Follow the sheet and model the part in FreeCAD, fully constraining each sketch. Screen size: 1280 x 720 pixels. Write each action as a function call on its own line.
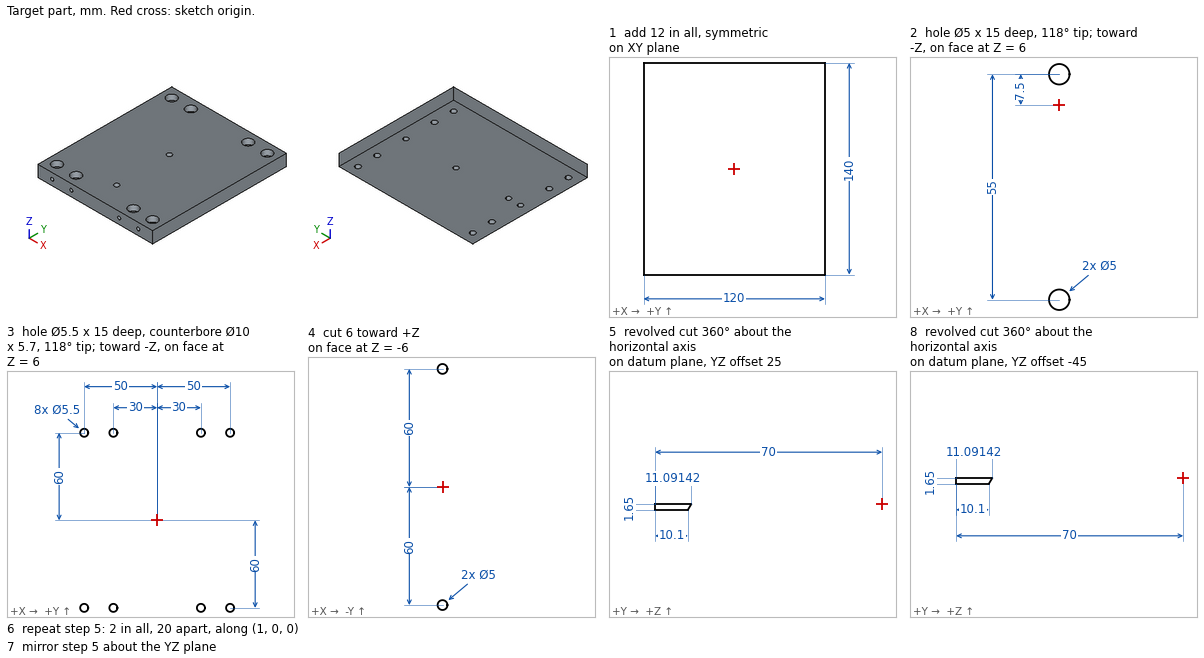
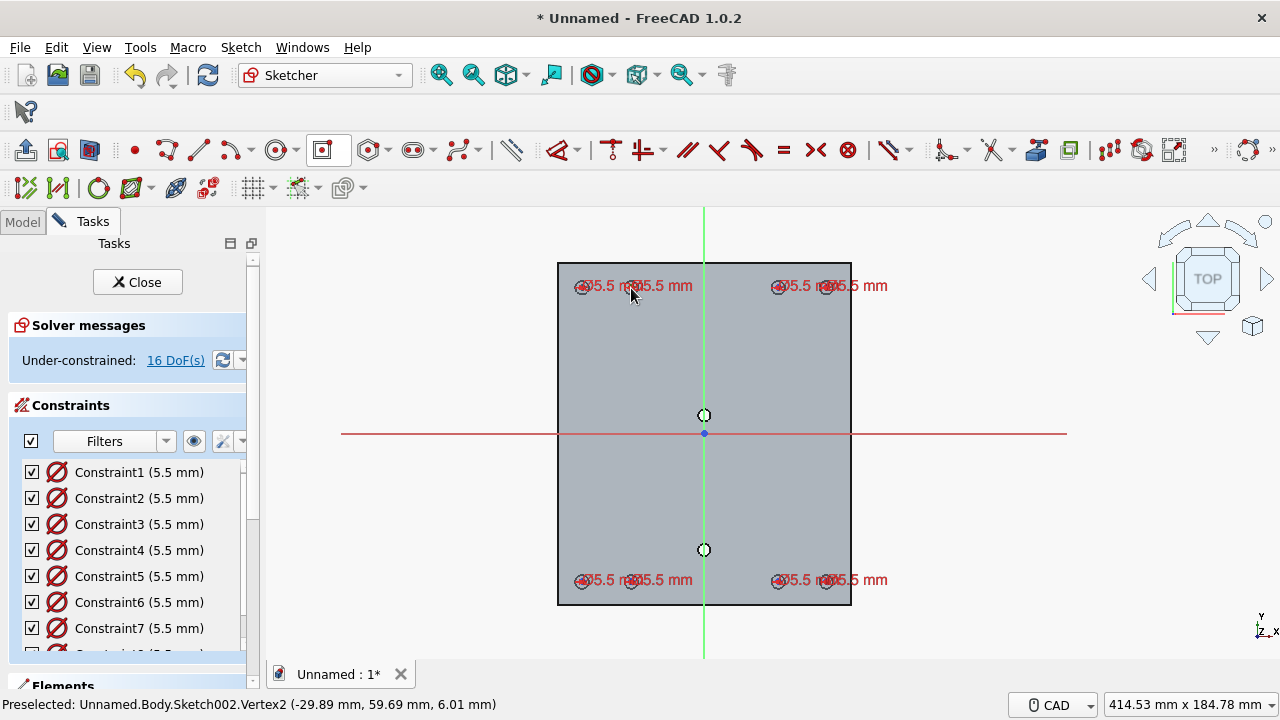
key(h)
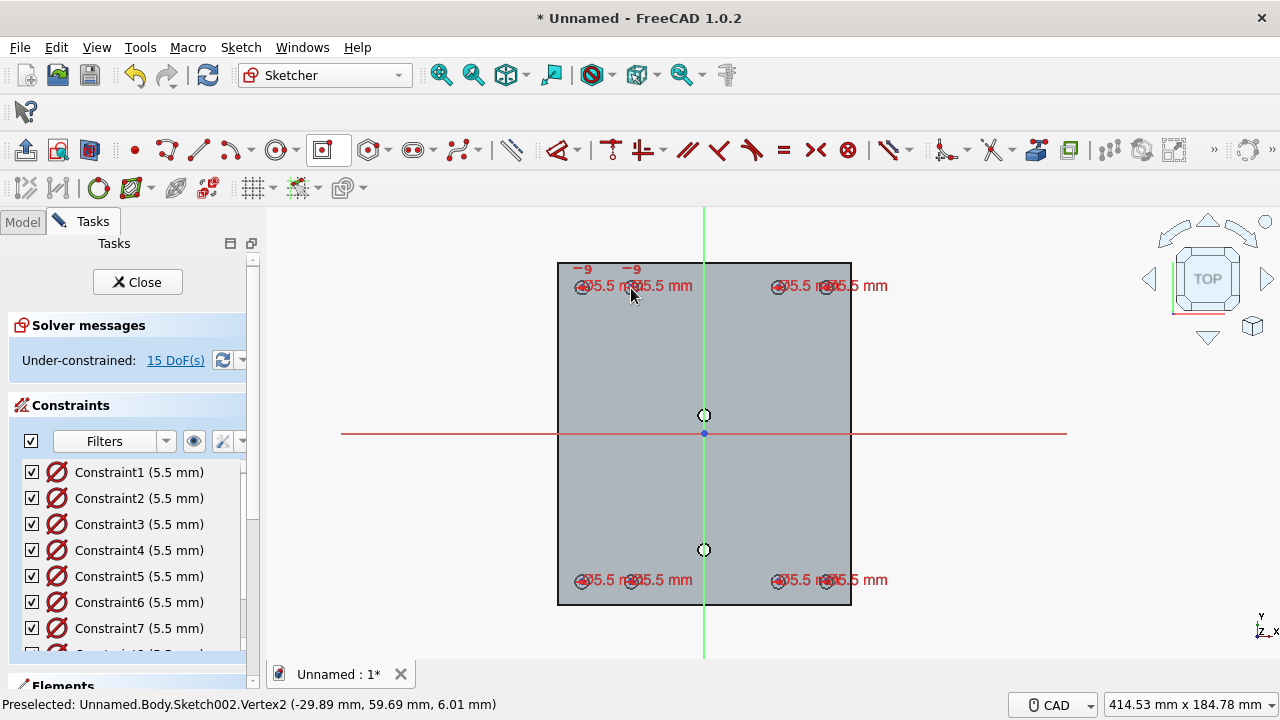
click(631, 288)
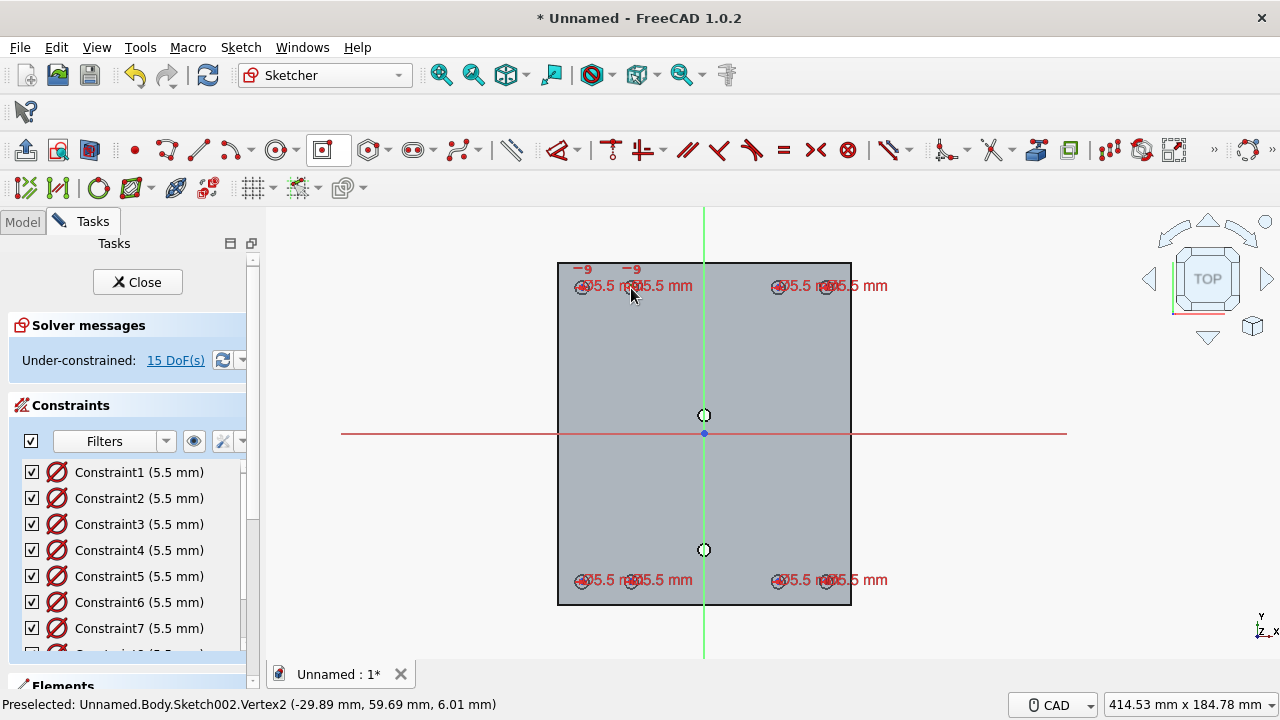
click(778, 288)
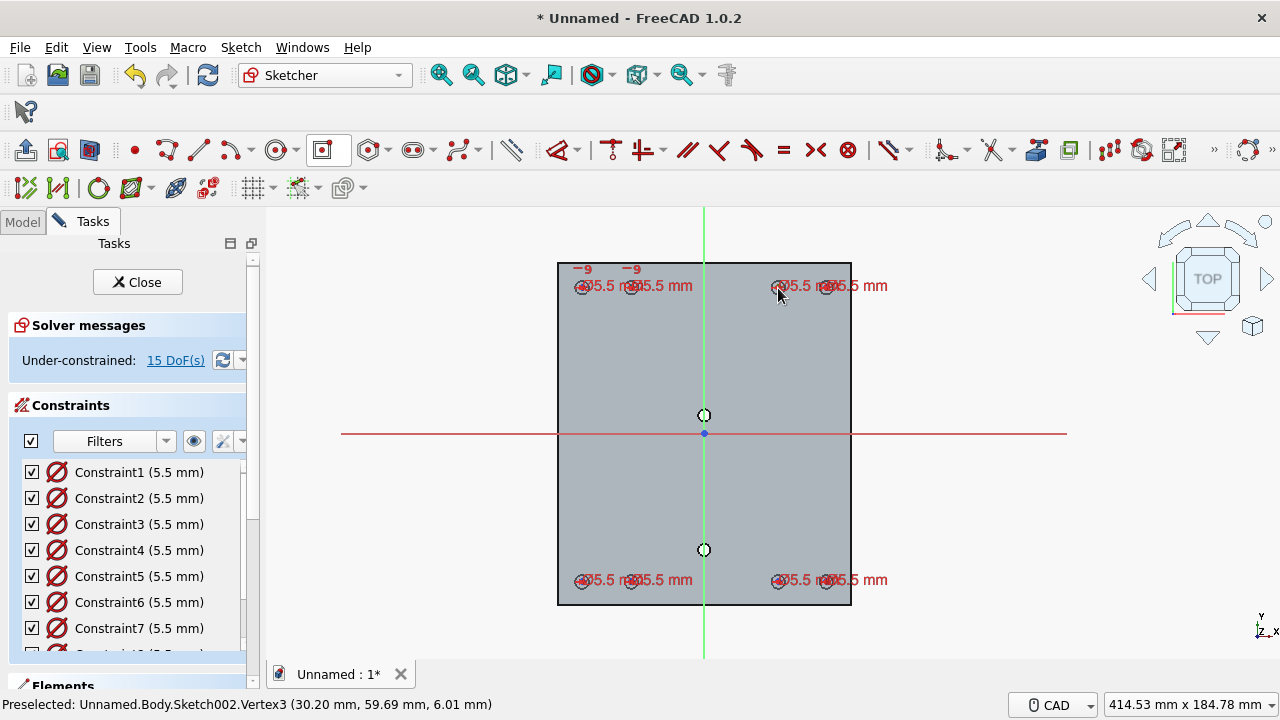
key(h)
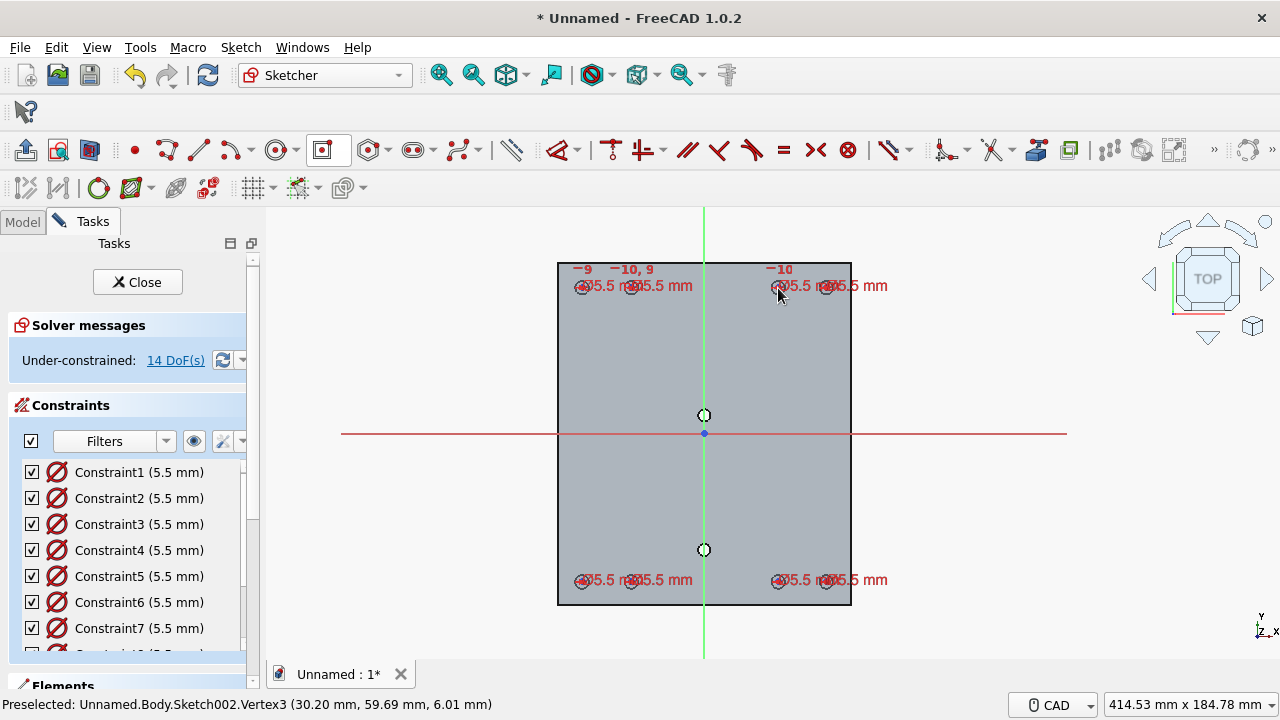
click(778, 288)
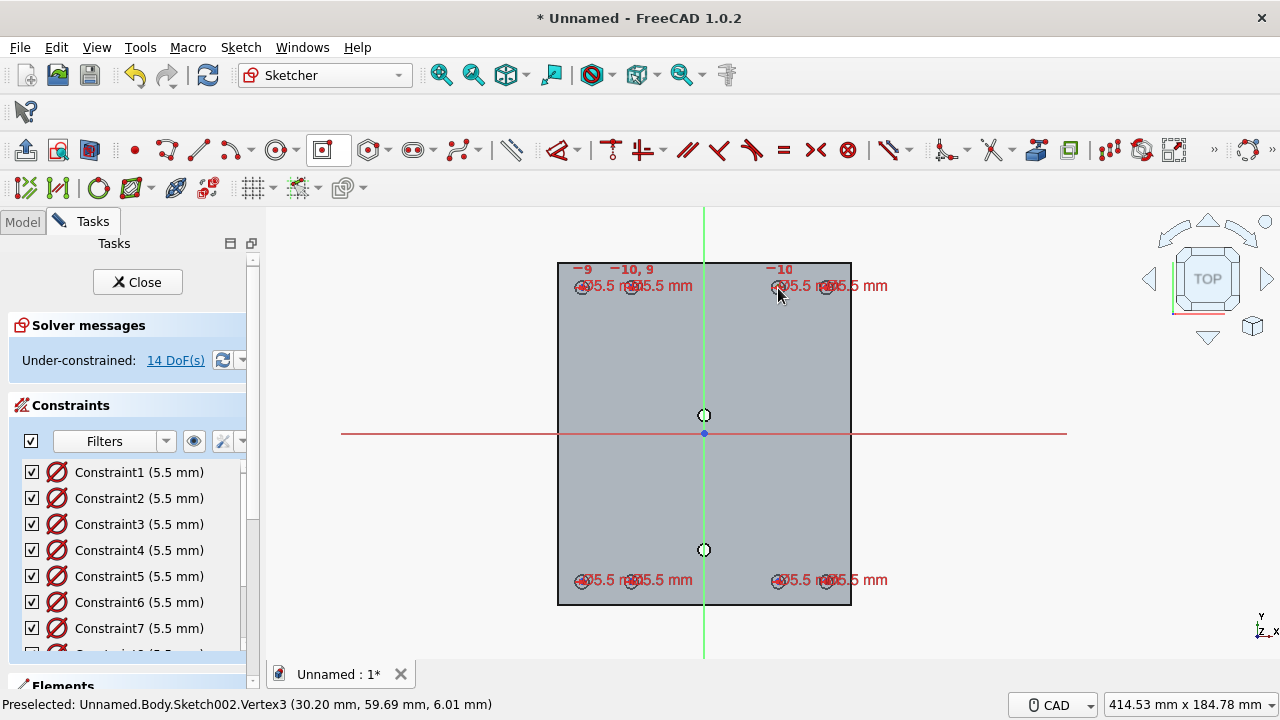
click(826, 288)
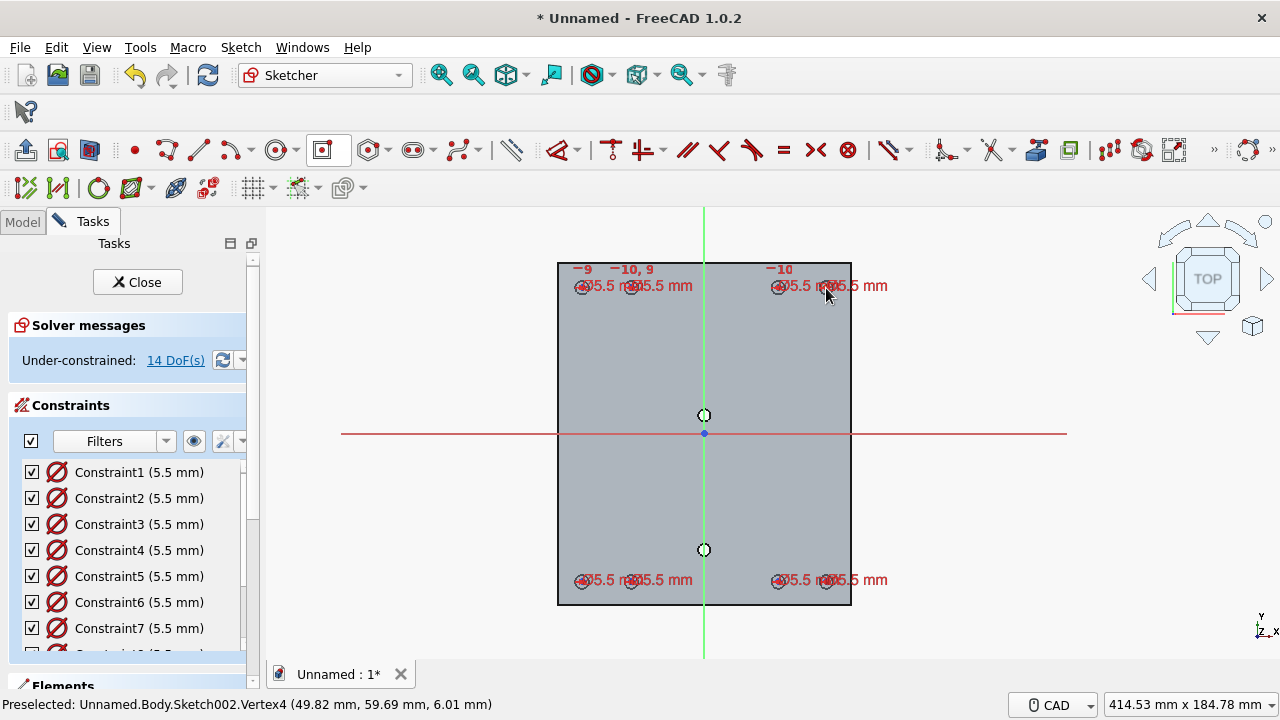
key(h)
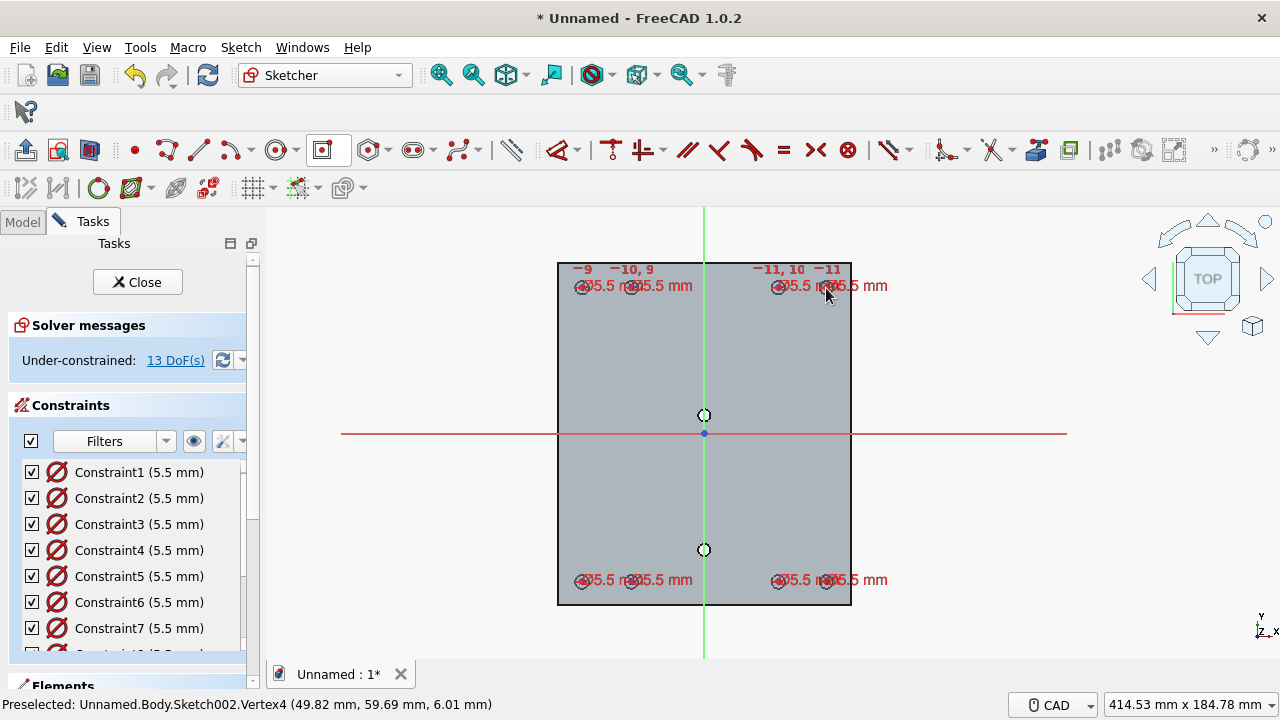
click(826, 288)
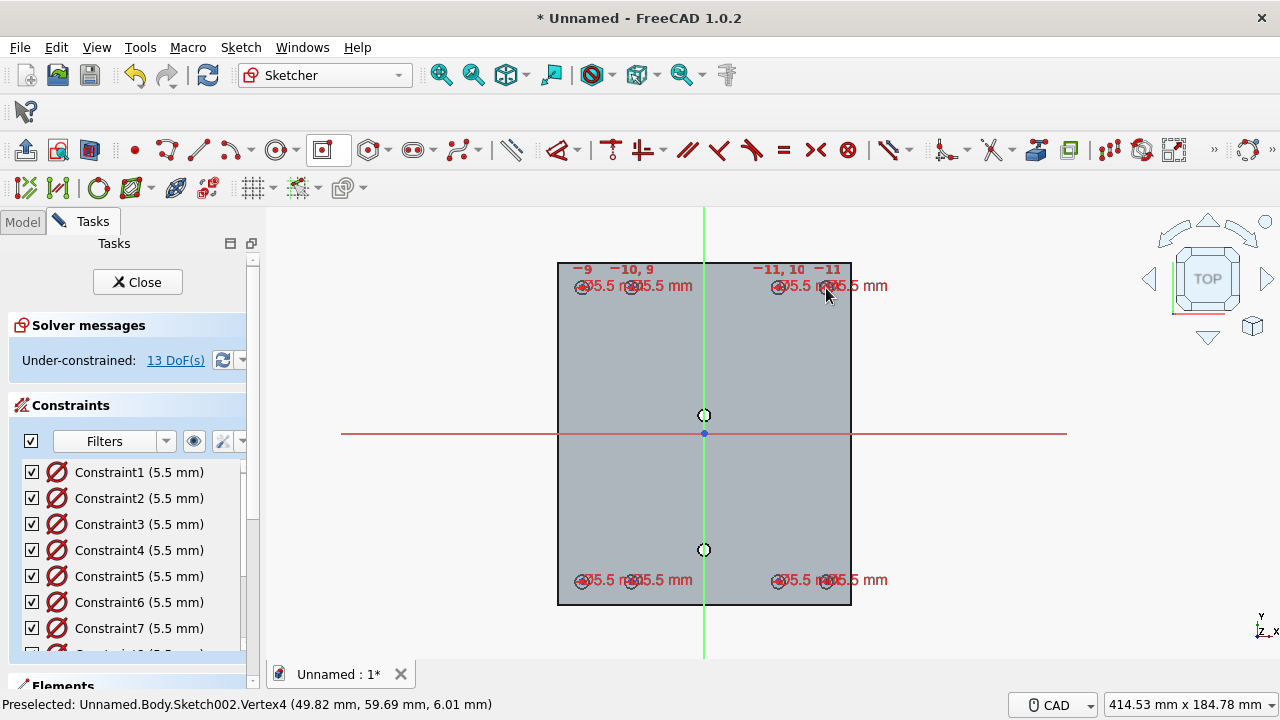
click(826, 582)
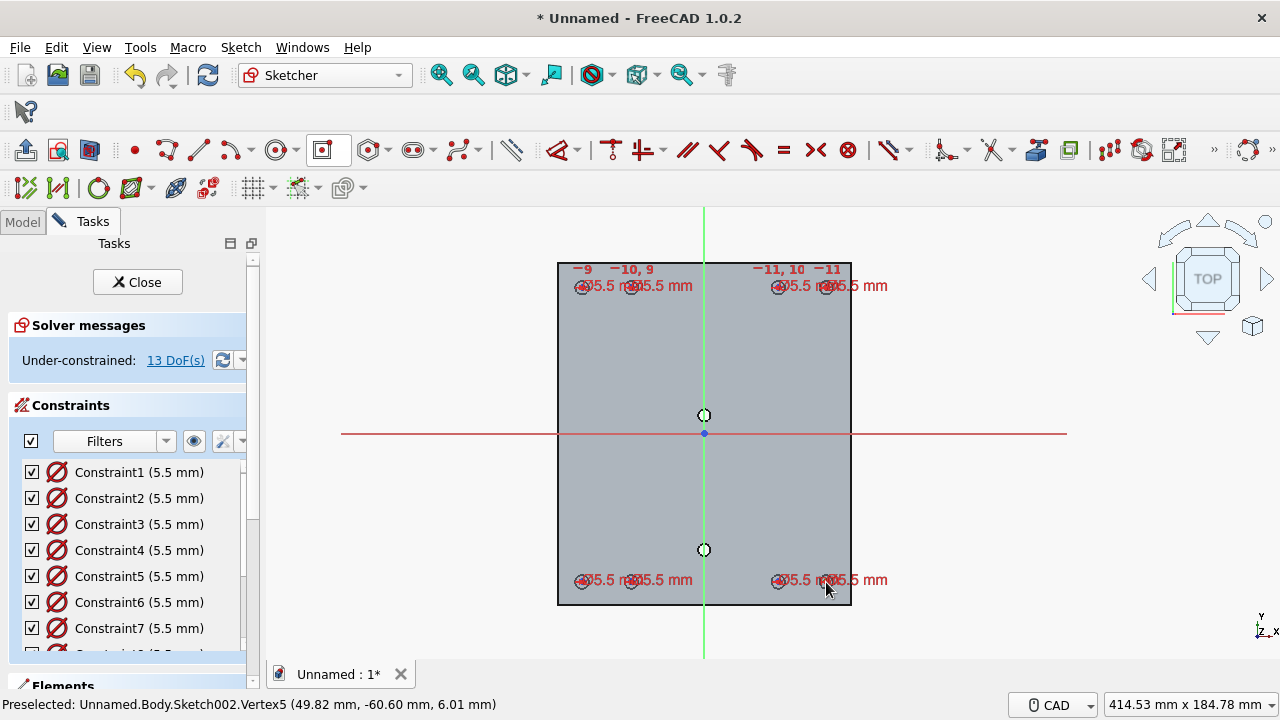
key(v)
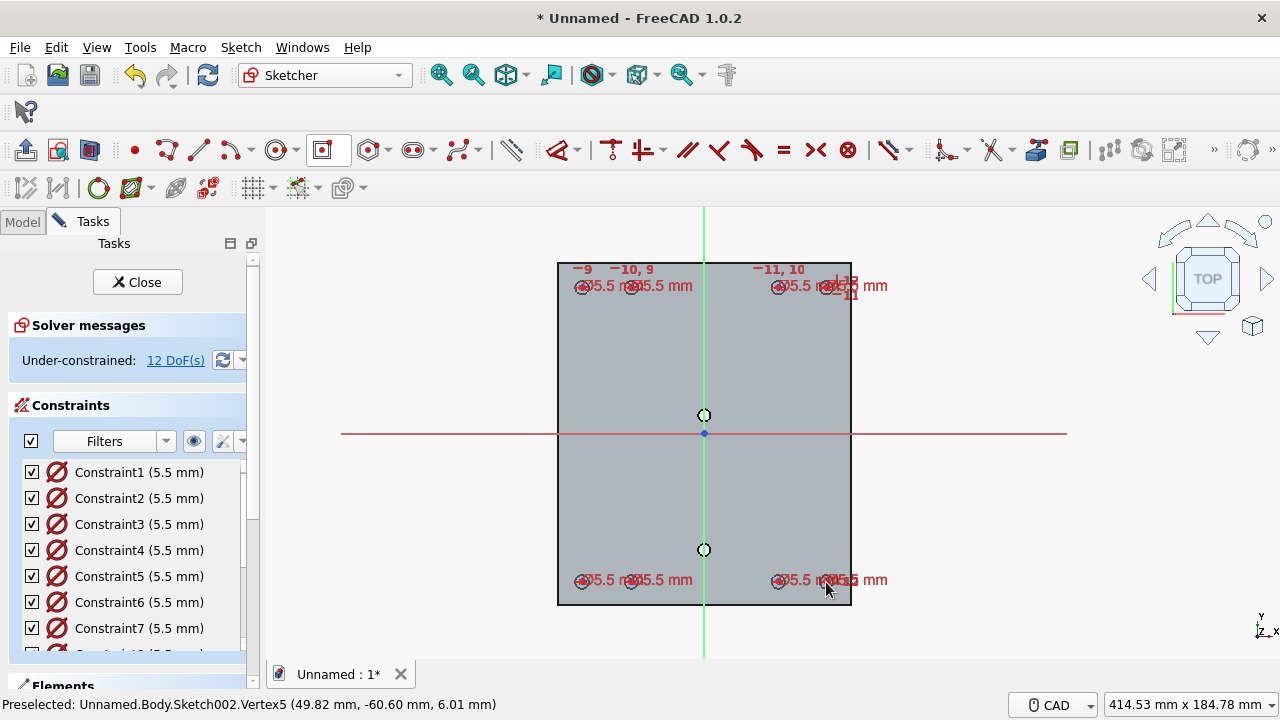
click(778, 288)